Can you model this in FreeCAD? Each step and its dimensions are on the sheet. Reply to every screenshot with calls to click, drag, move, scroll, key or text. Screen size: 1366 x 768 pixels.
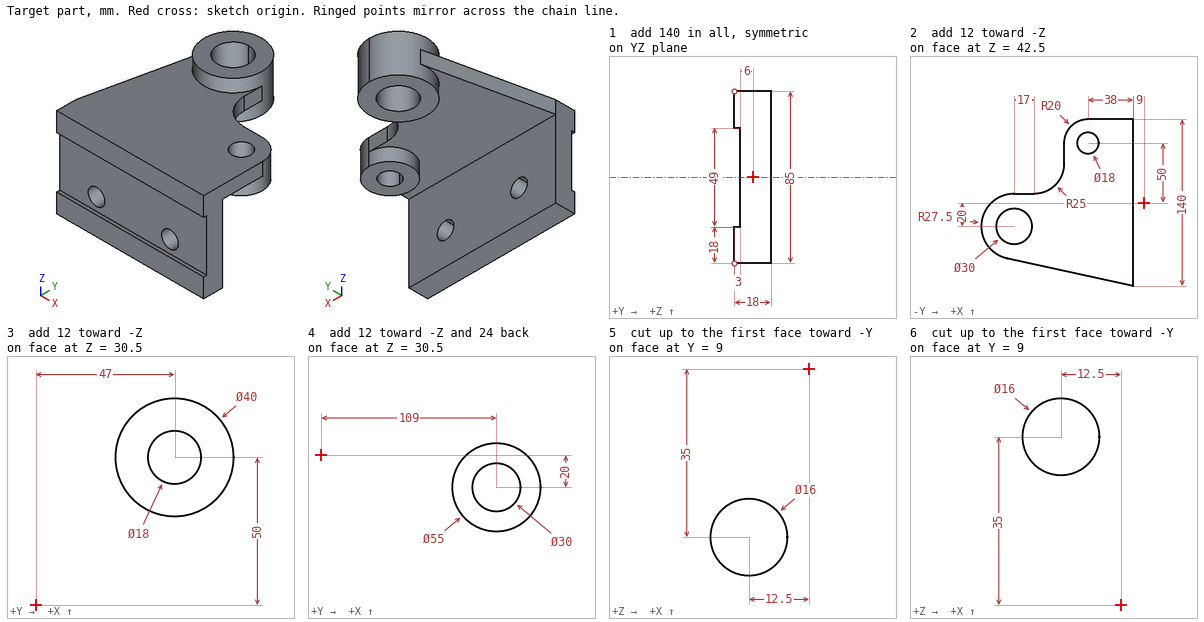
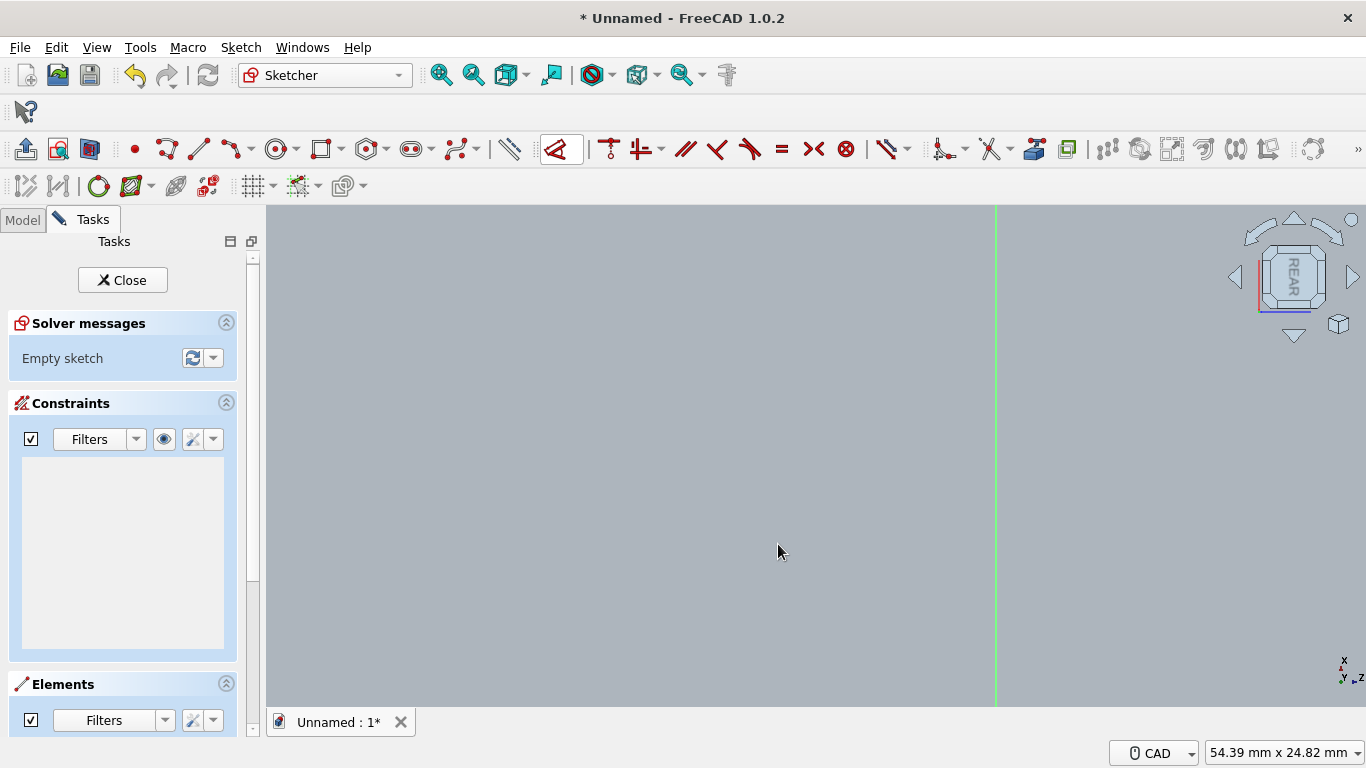
key(g)
key(c)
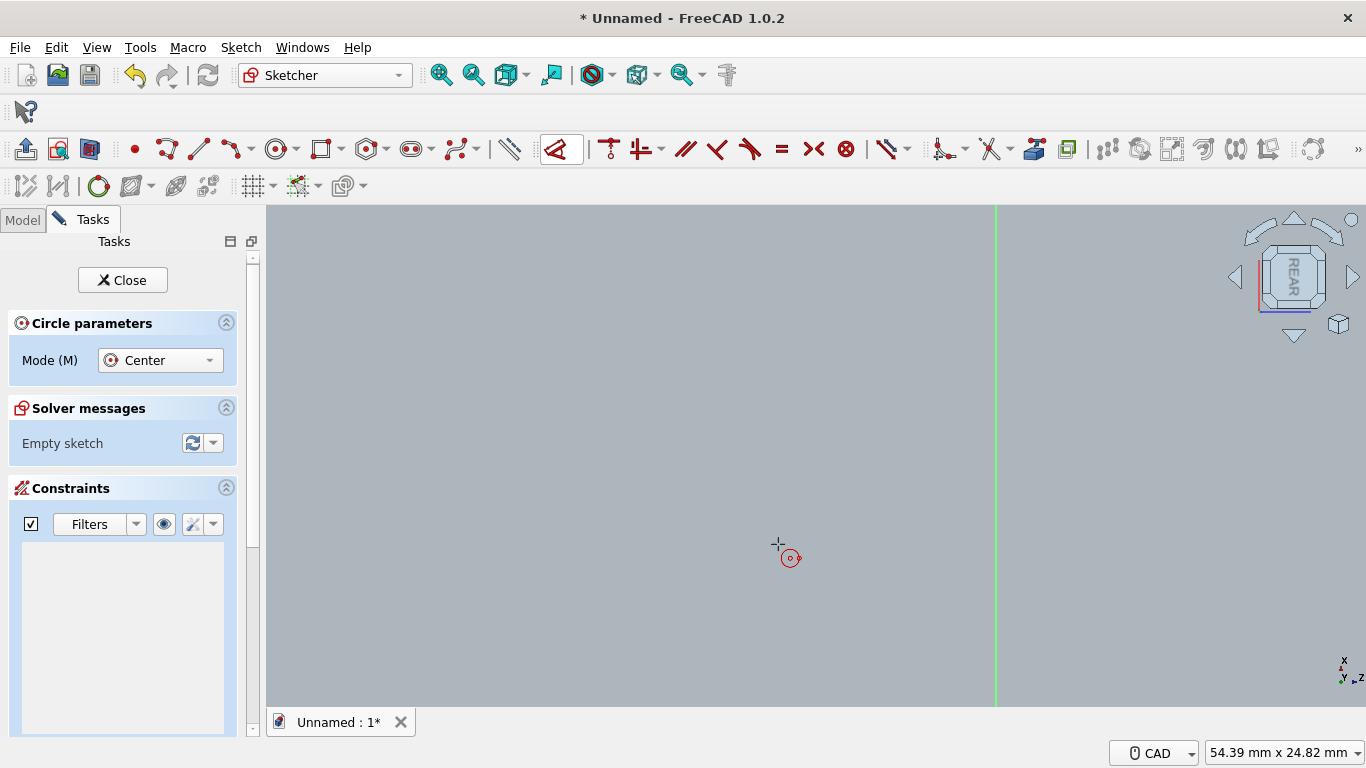
click(743, 452)
move(857, 338)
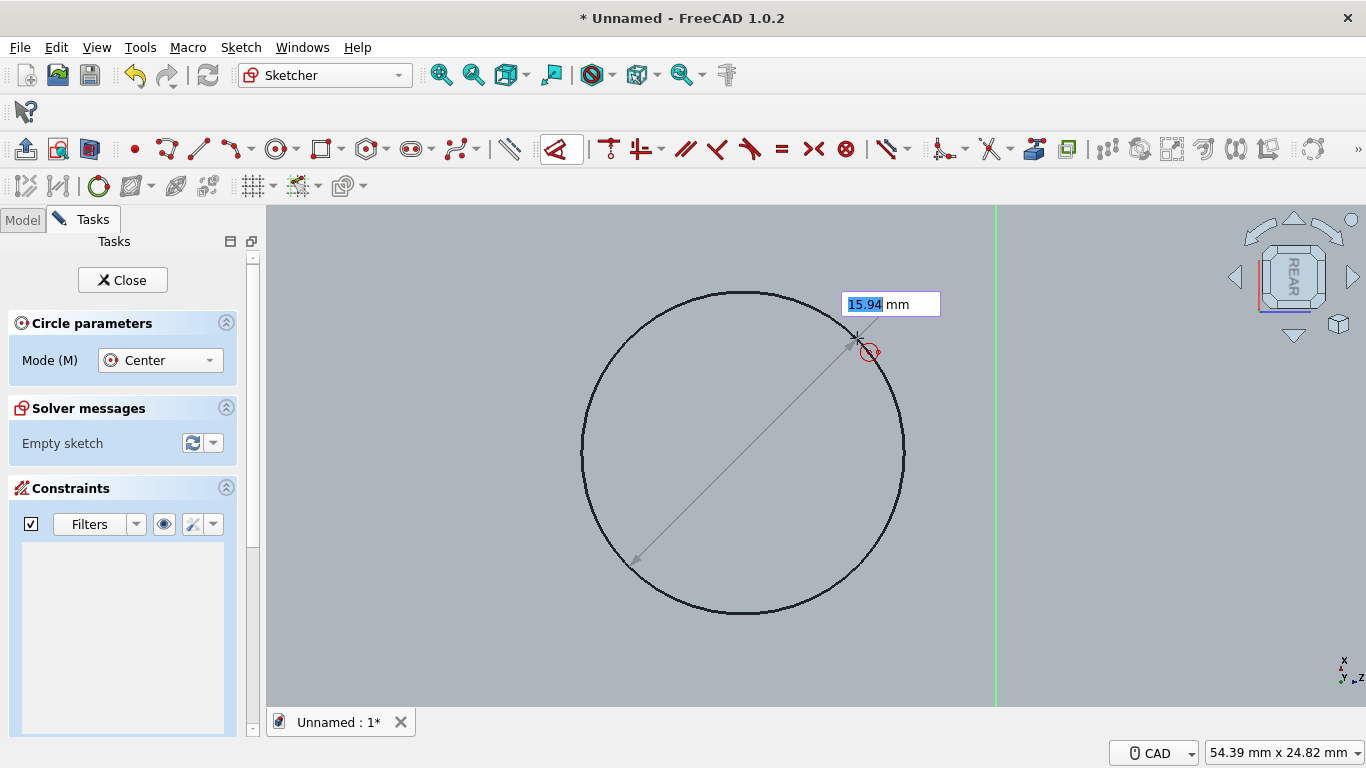
text(16)
key(Return)
key(Escape)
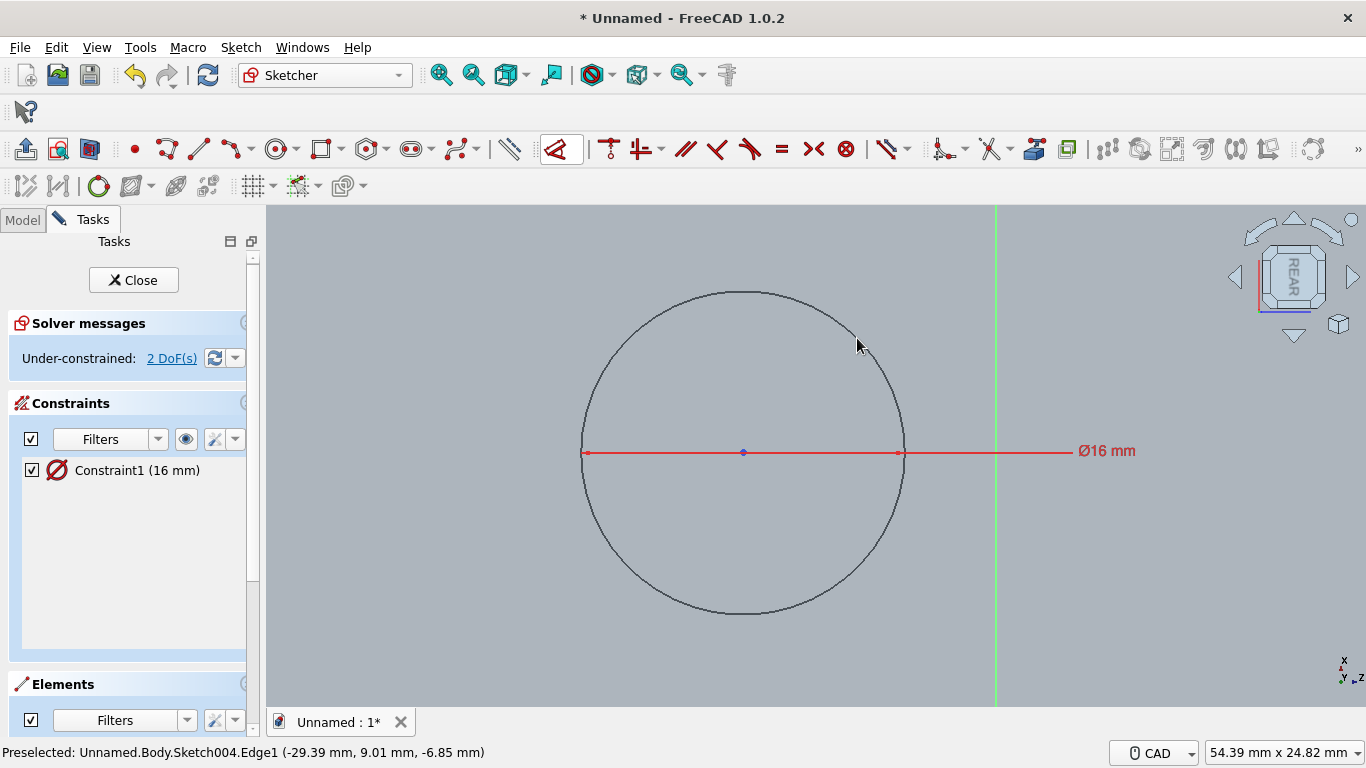
click(743, 453)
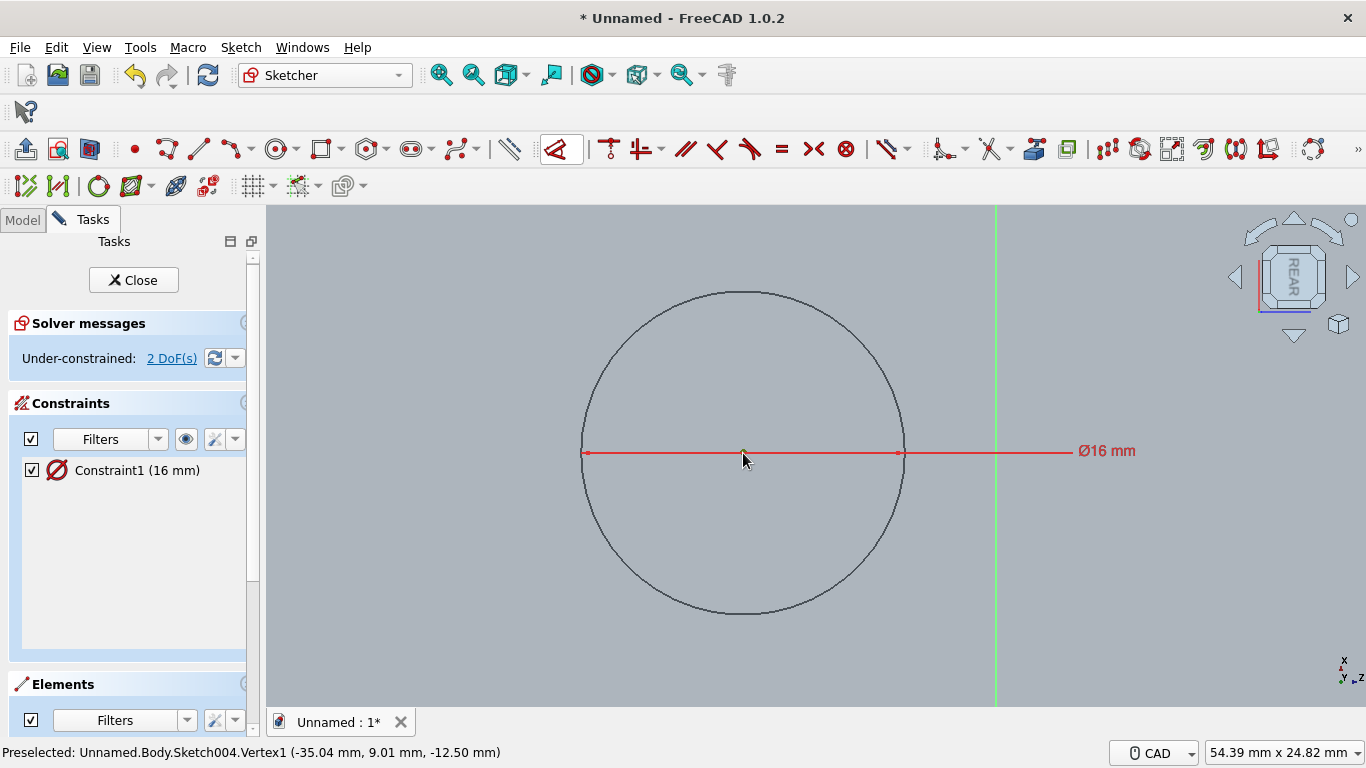
key(i)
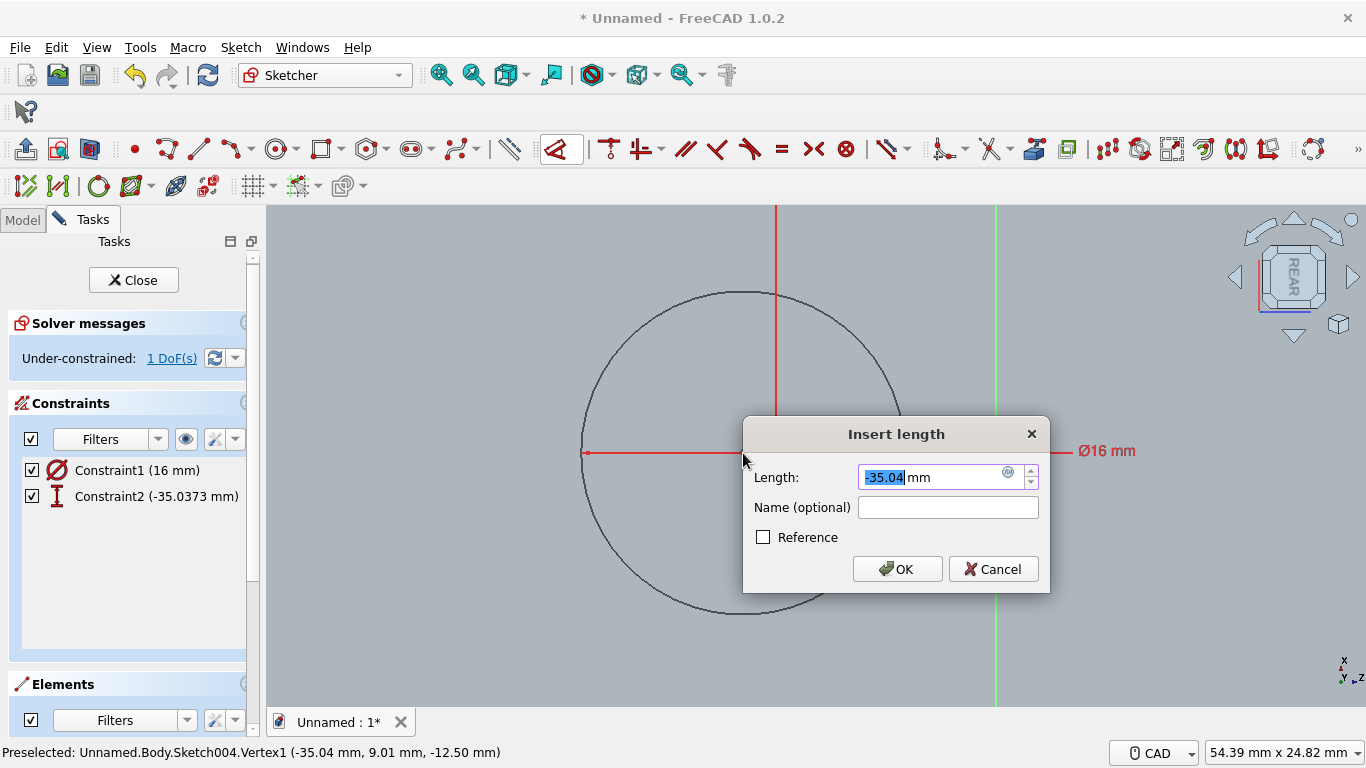
text(-35)
key(Return)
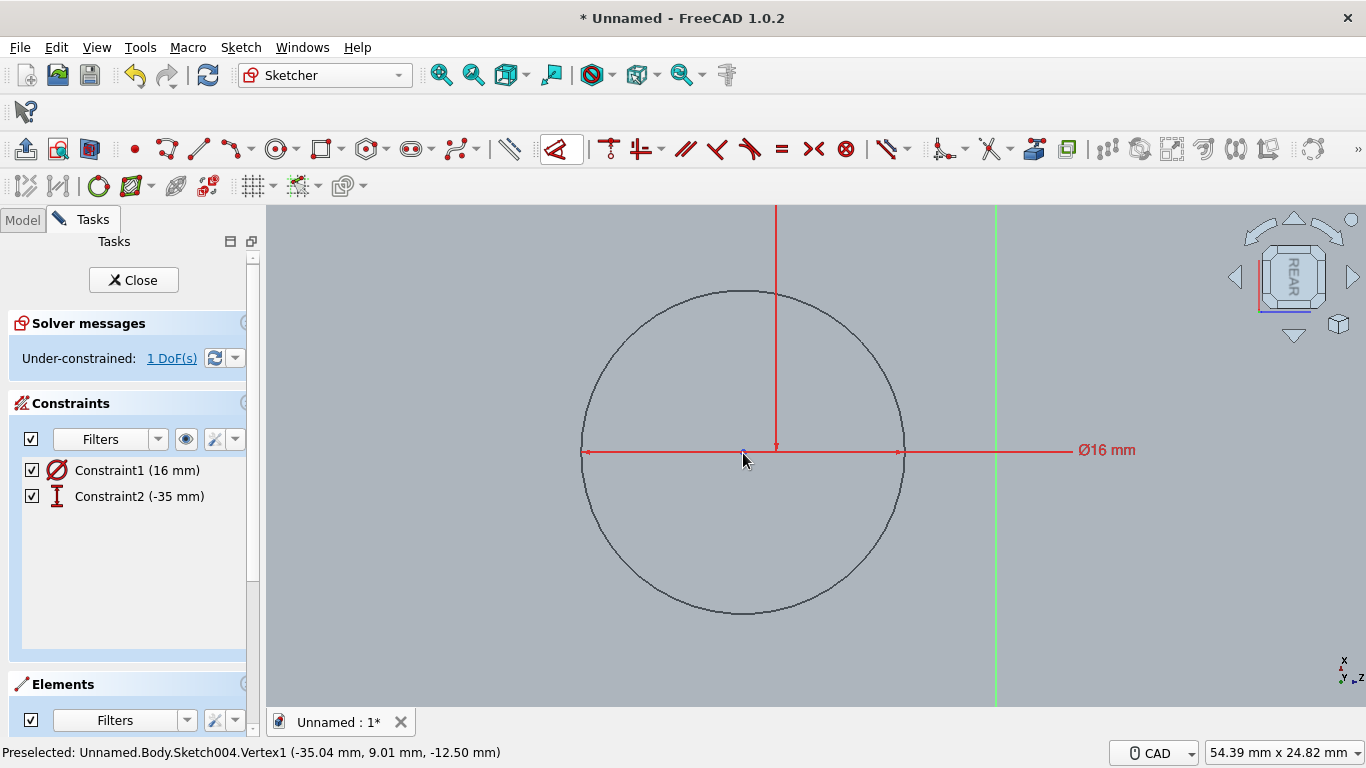
click(743, 452)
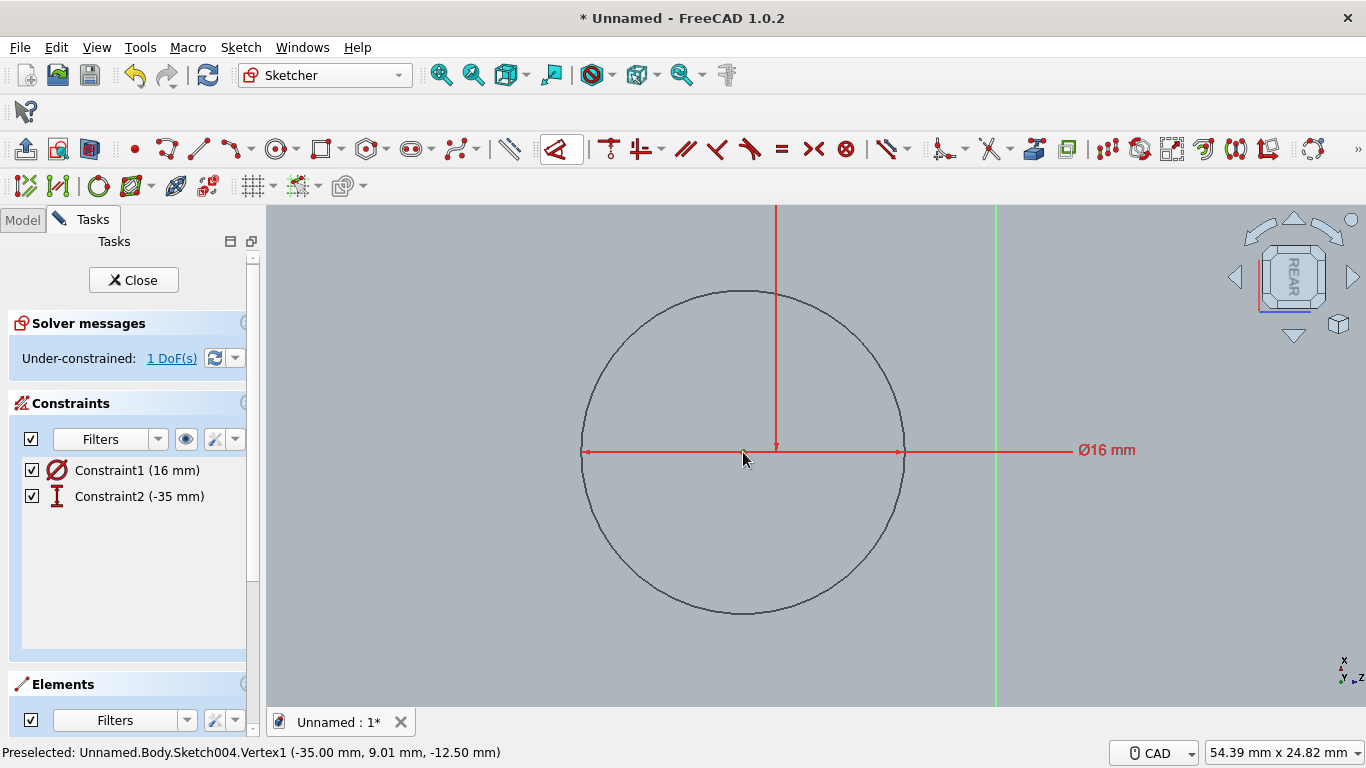
key(l)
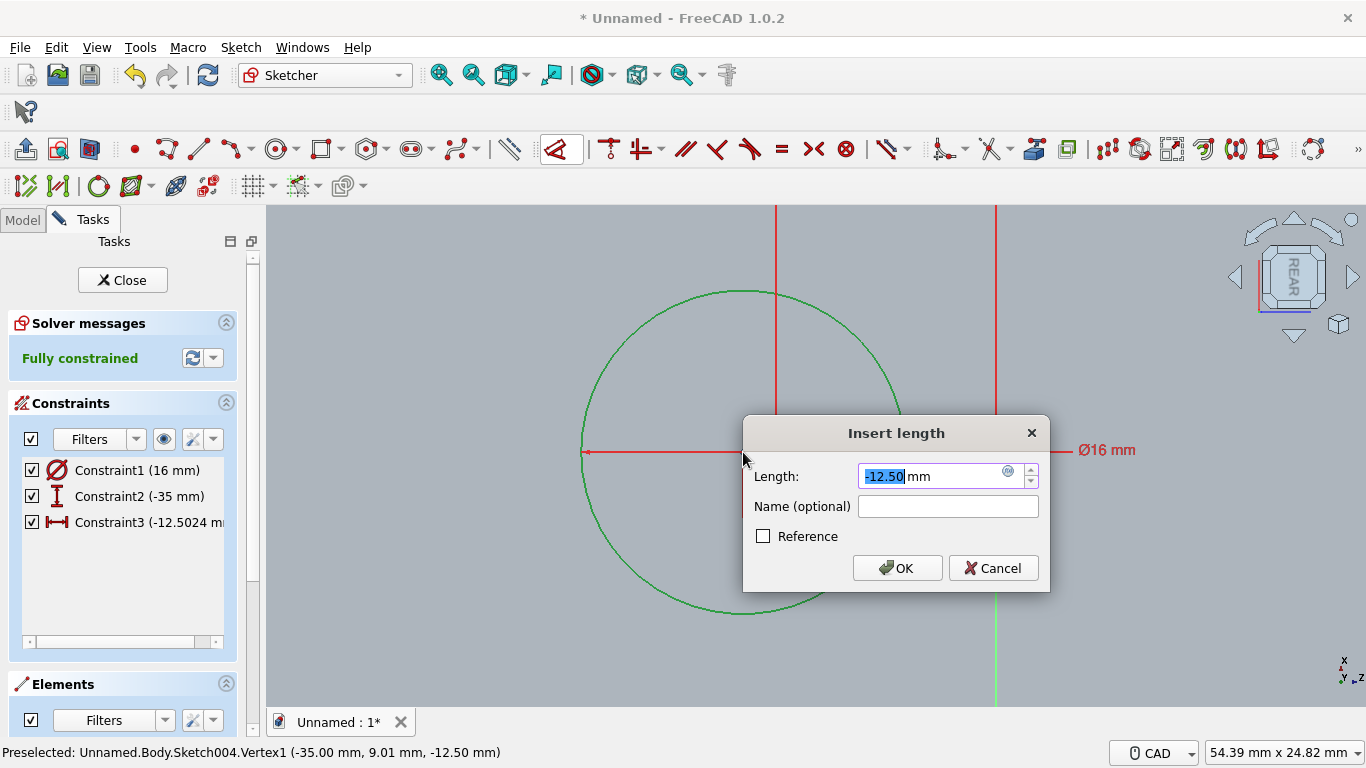
text(-12.5)
key(Return)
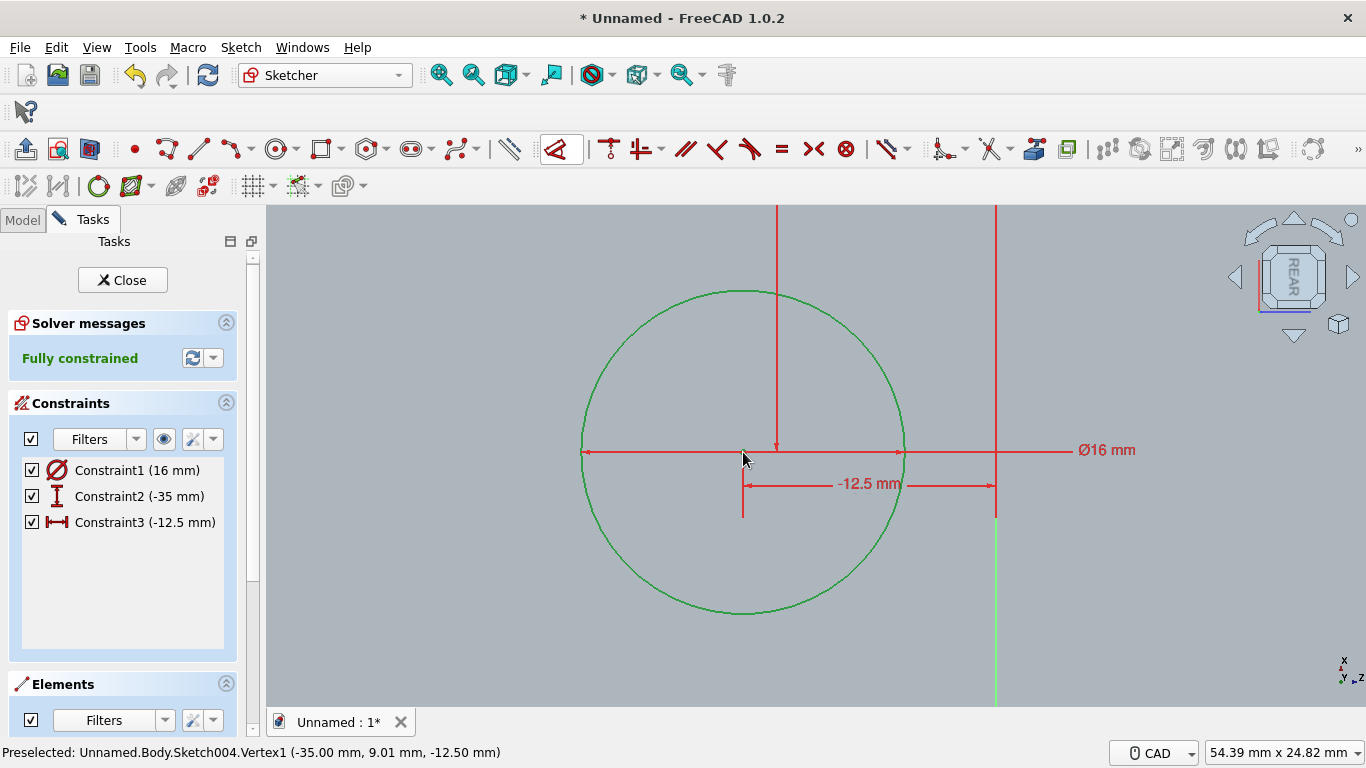
click(123, 280)